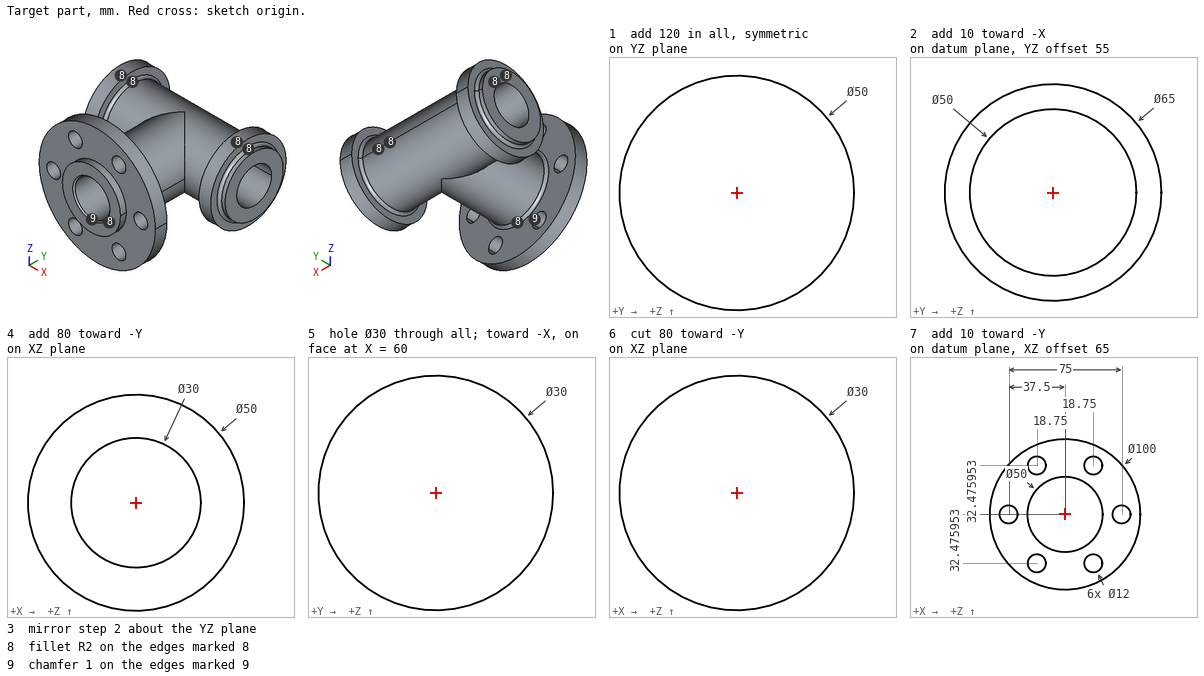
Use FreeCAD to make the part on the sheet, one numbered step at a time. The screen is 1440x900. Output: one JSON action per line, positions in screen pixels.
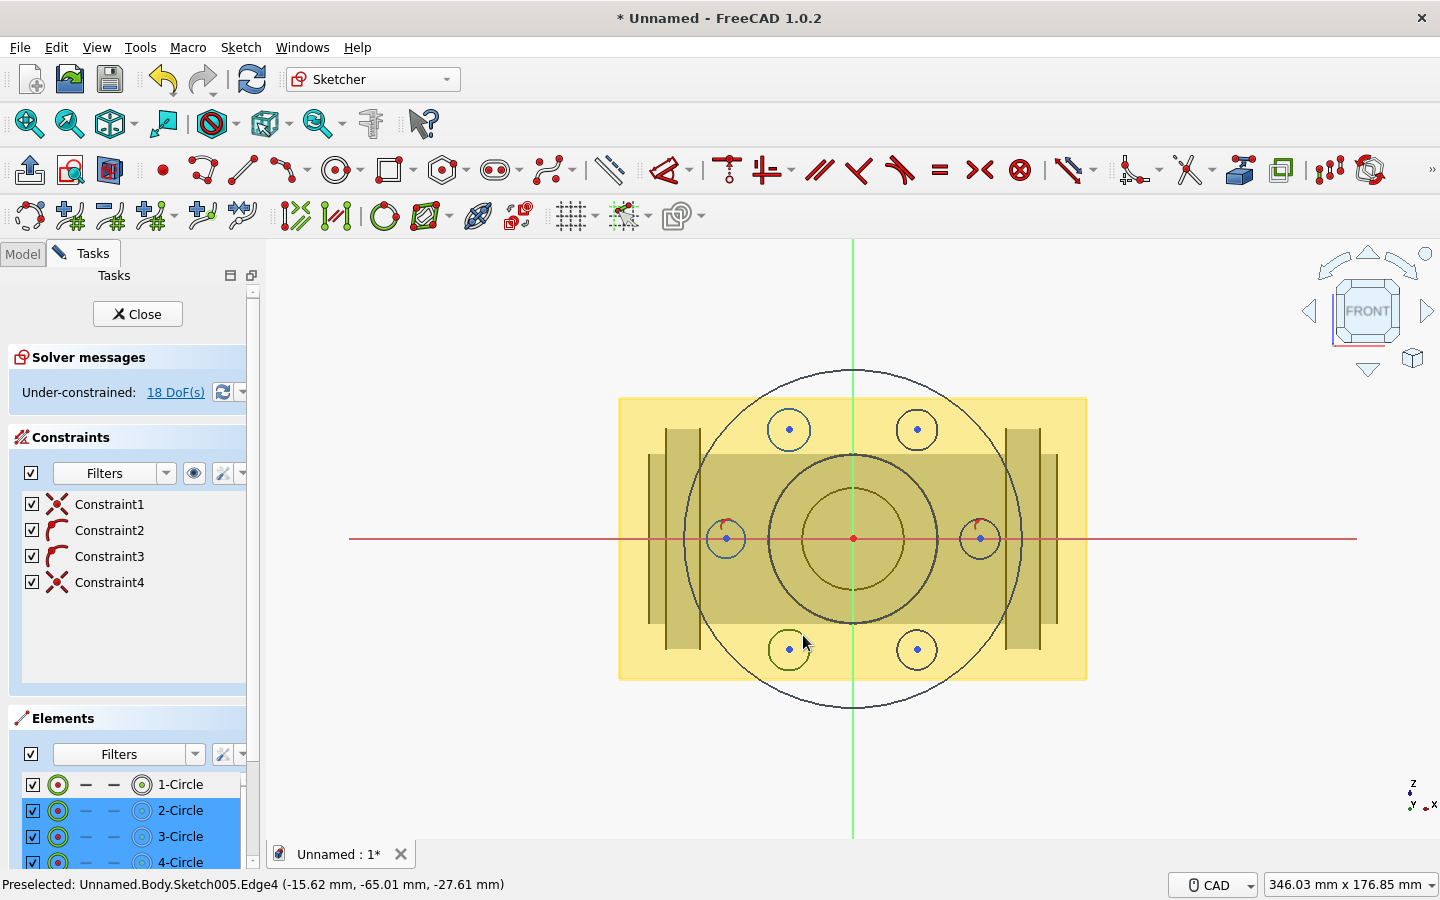
{"action": "left_click", "coordinate": [931, 415]}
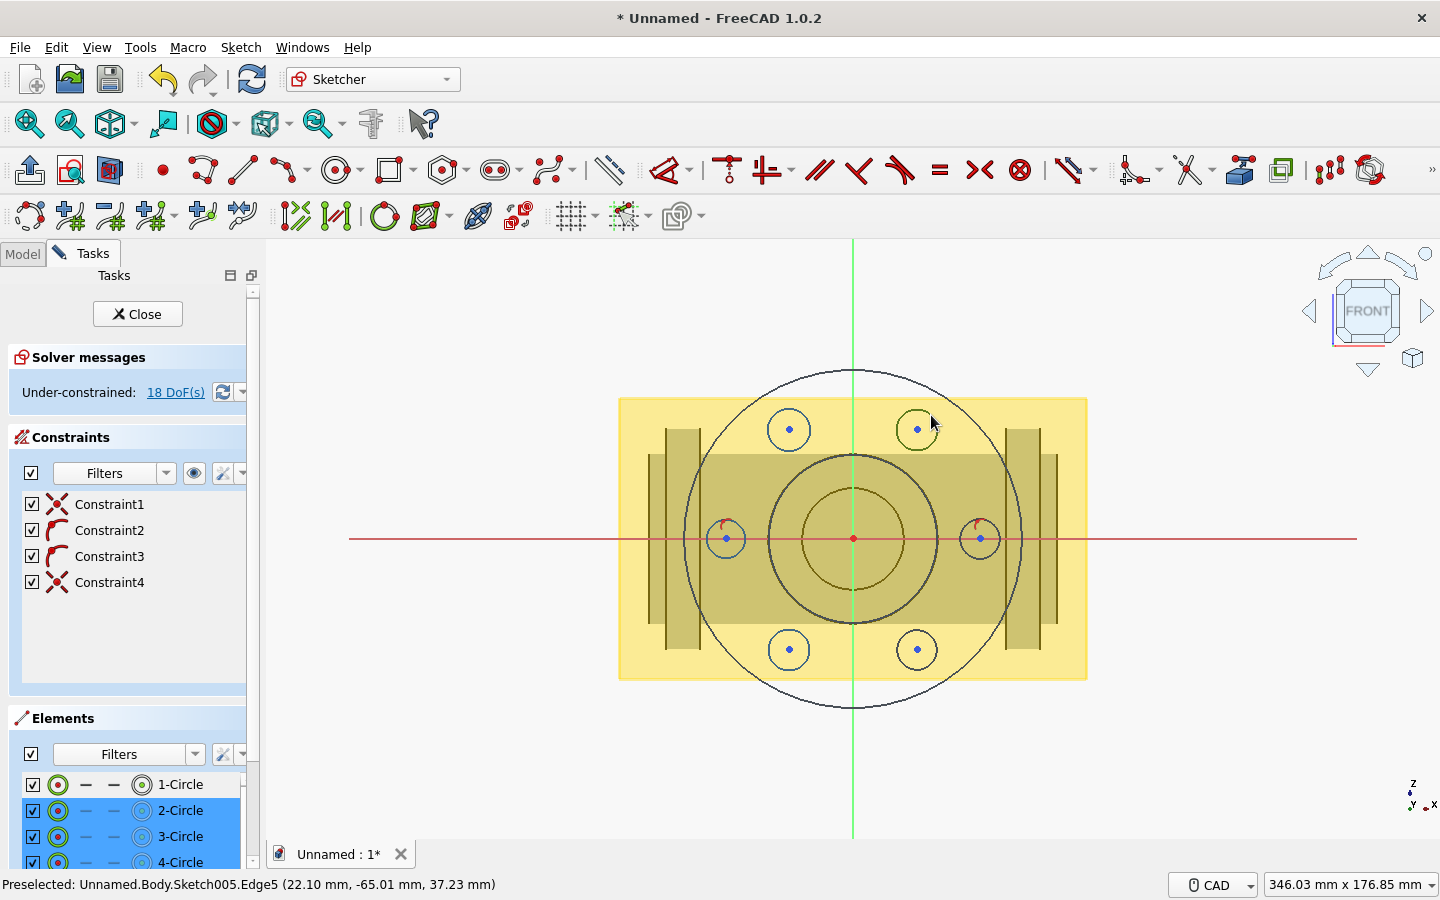
{"action": "left_click", "coordinate": [994, 525]}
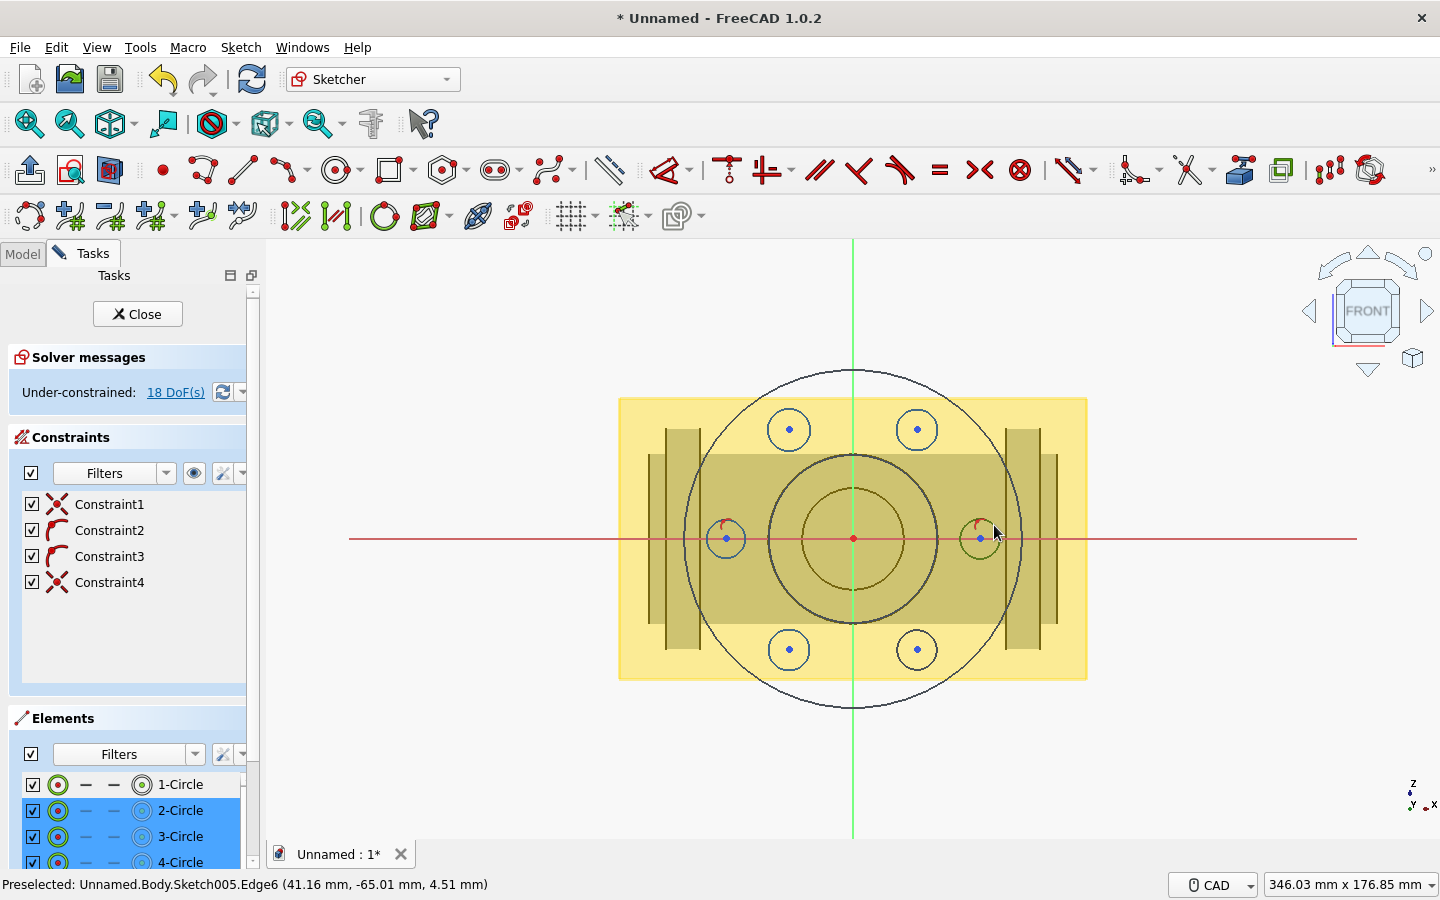
{"action": "left_click", "coordinate": [931, 636]}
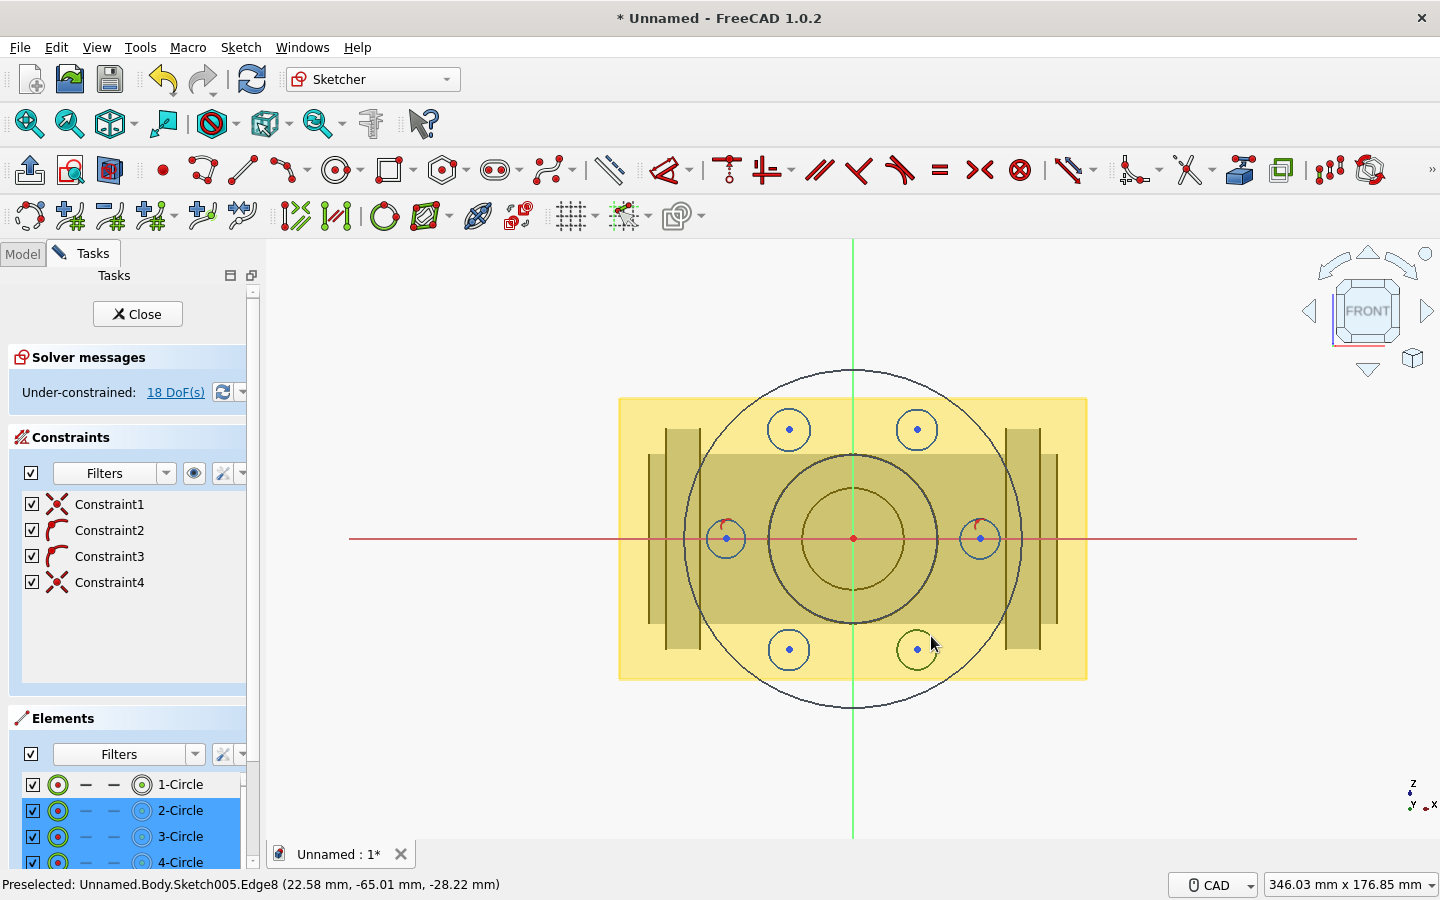
{"action": "key", "text": "e"}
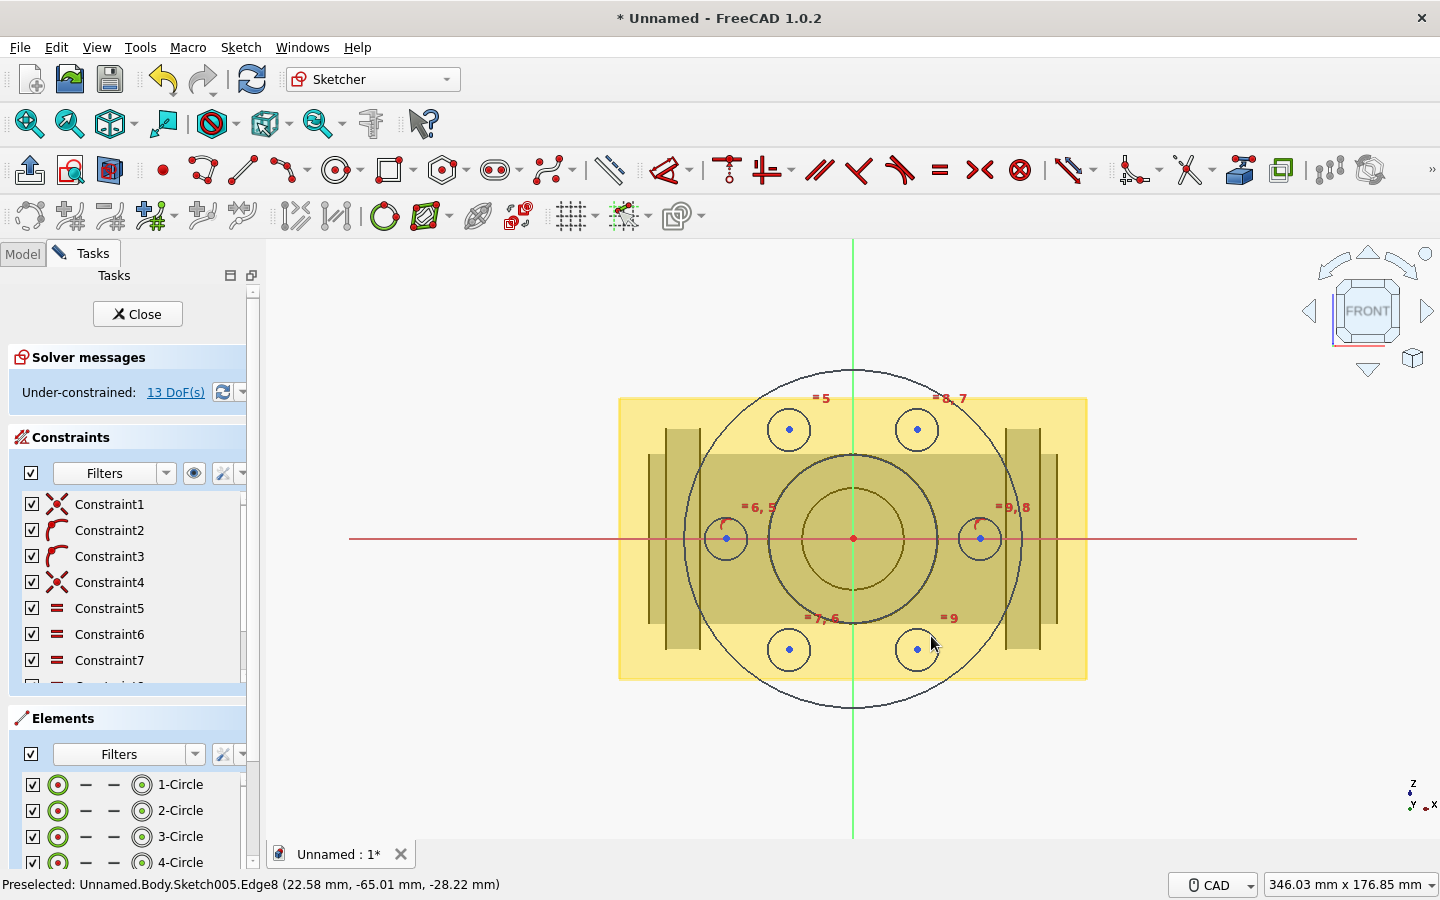
{"action": "left_click", "coordinate": [789, 430]}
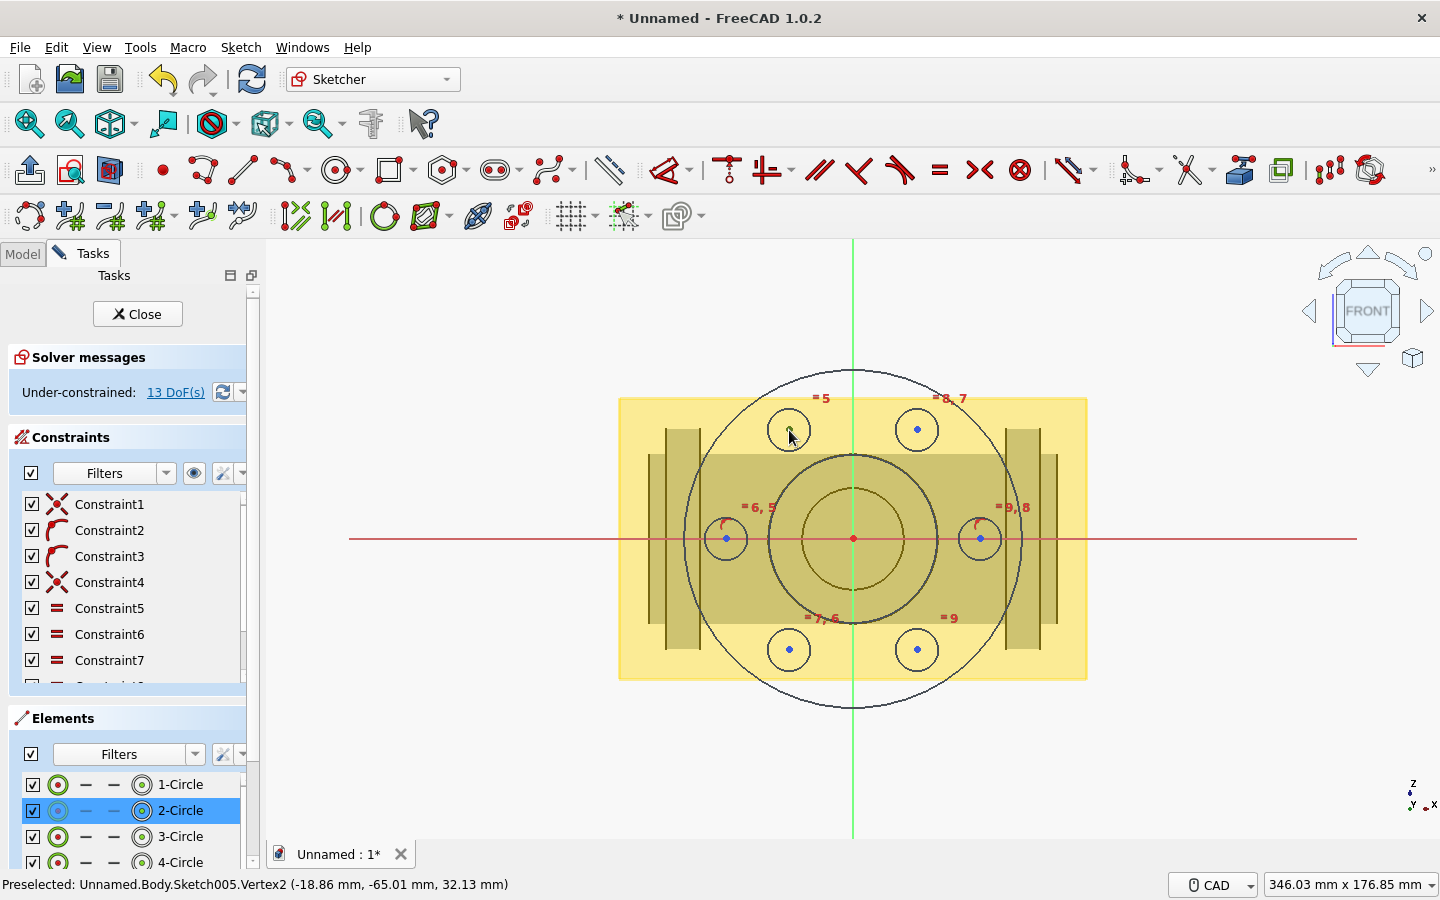
{"action": "left_click", "coordinate": [789, 650]}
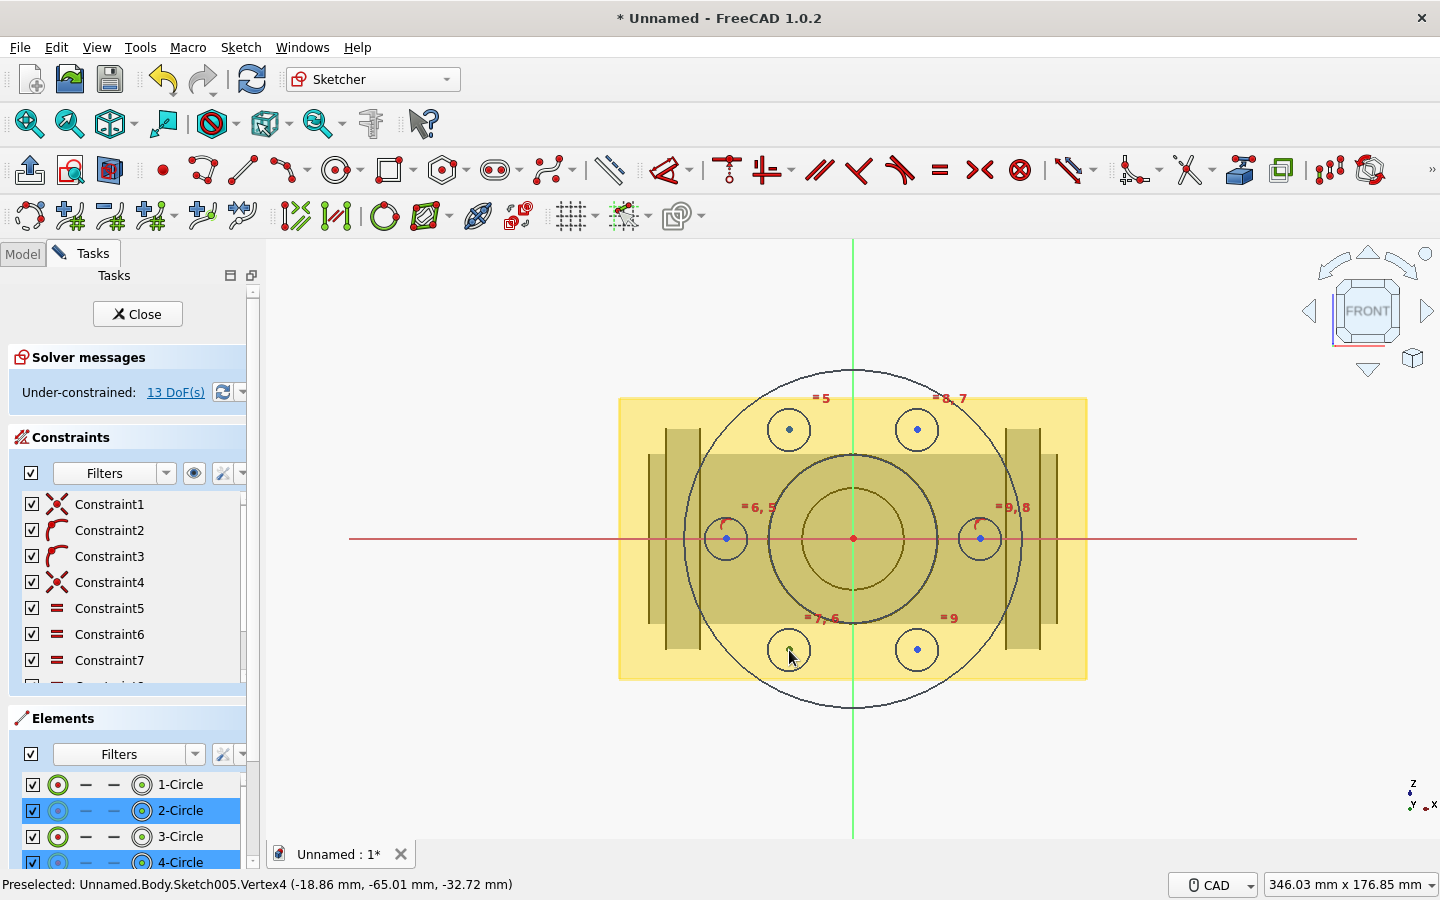
{"action": "key", "text": "v"}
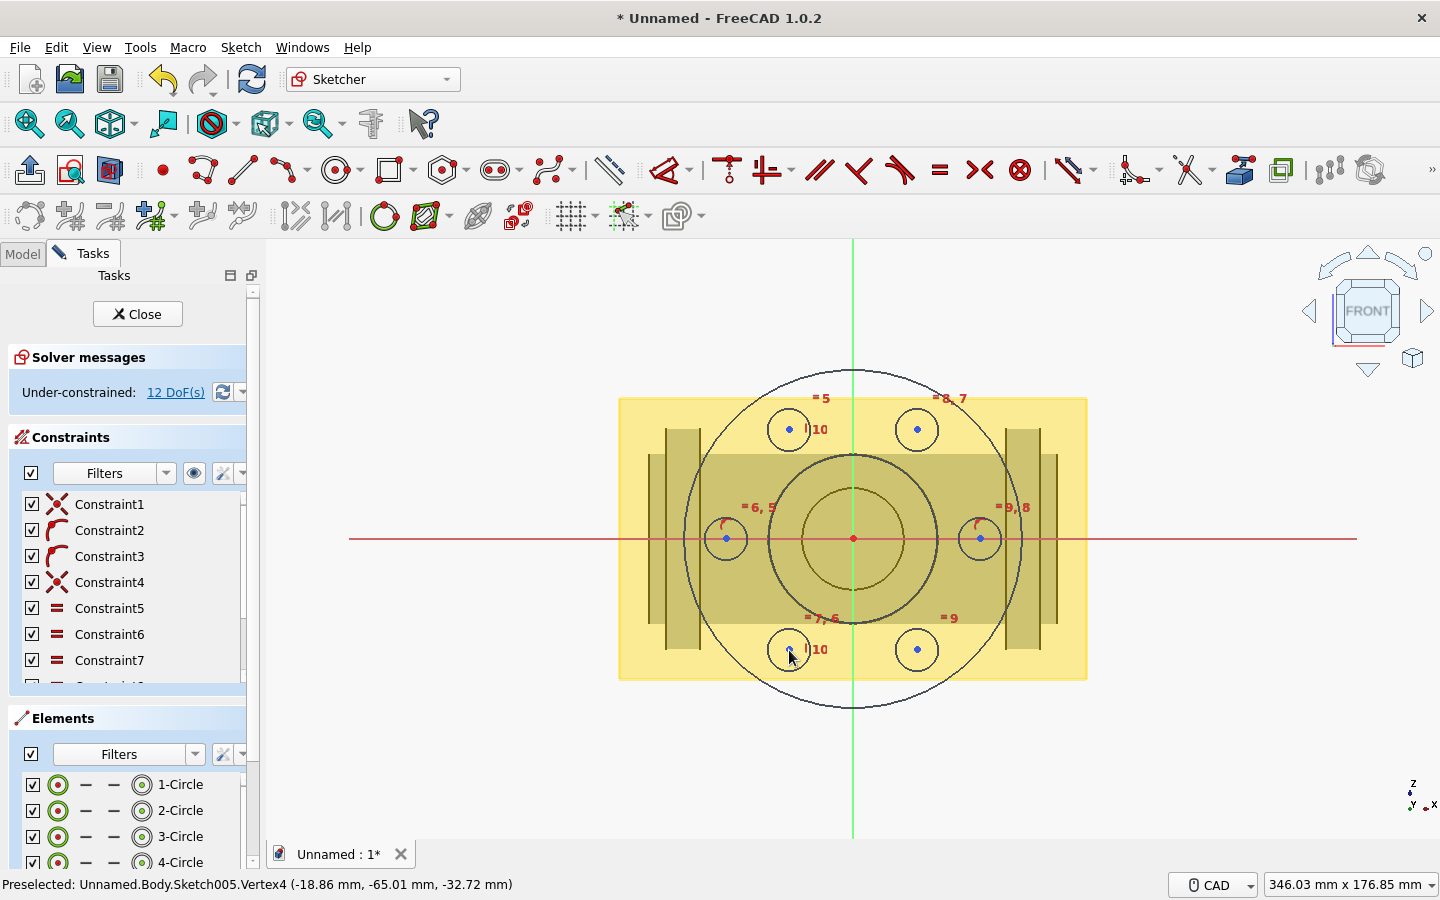
{"action": "left_click", "coordinate": [789, 430]}